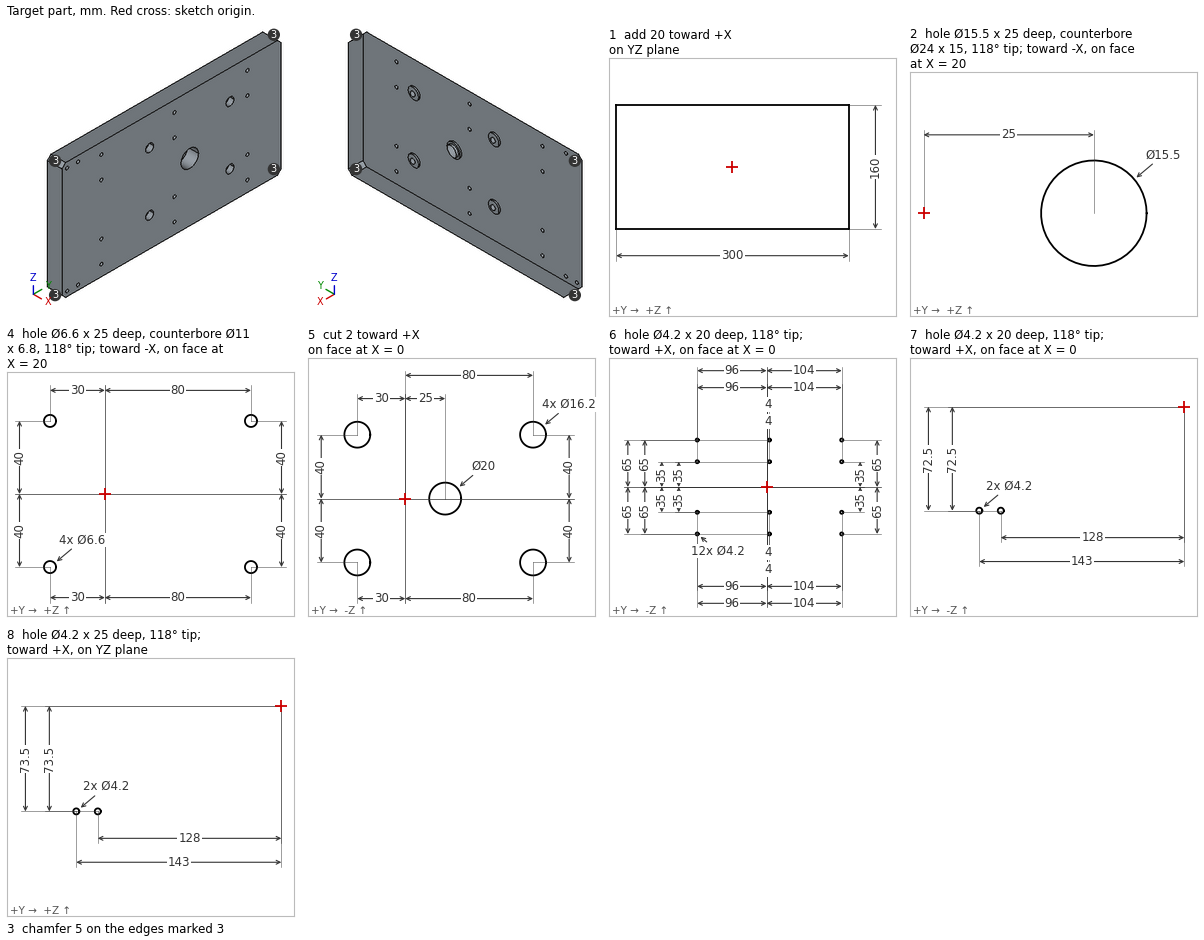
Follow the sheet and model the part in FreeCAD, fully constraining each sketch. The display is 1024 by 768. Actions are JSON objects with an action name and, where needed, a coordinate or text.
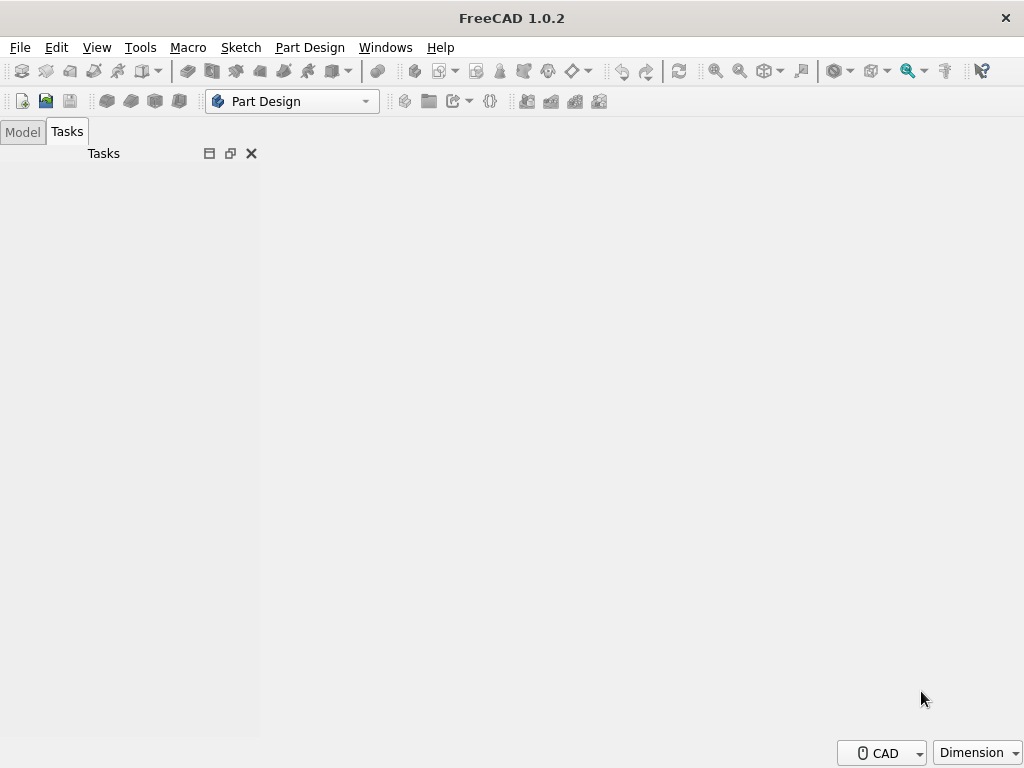
{"action": "left_click", "coordinate": [22, 102]}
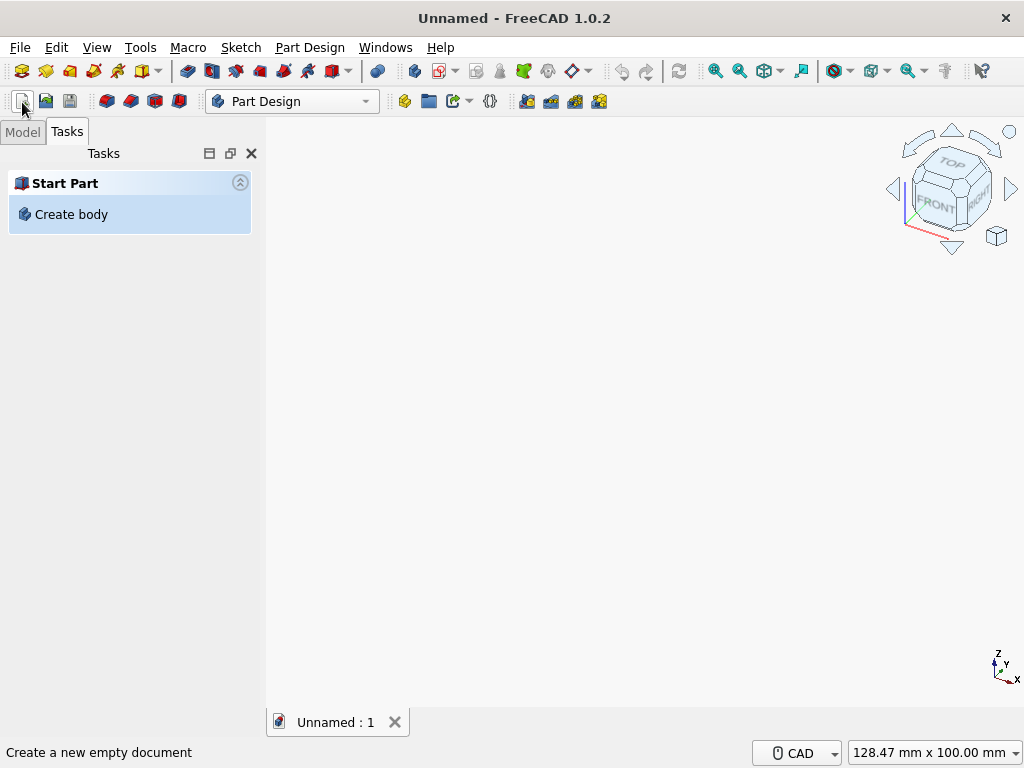
{"action": "left_click", "coordinate": [440, 72]}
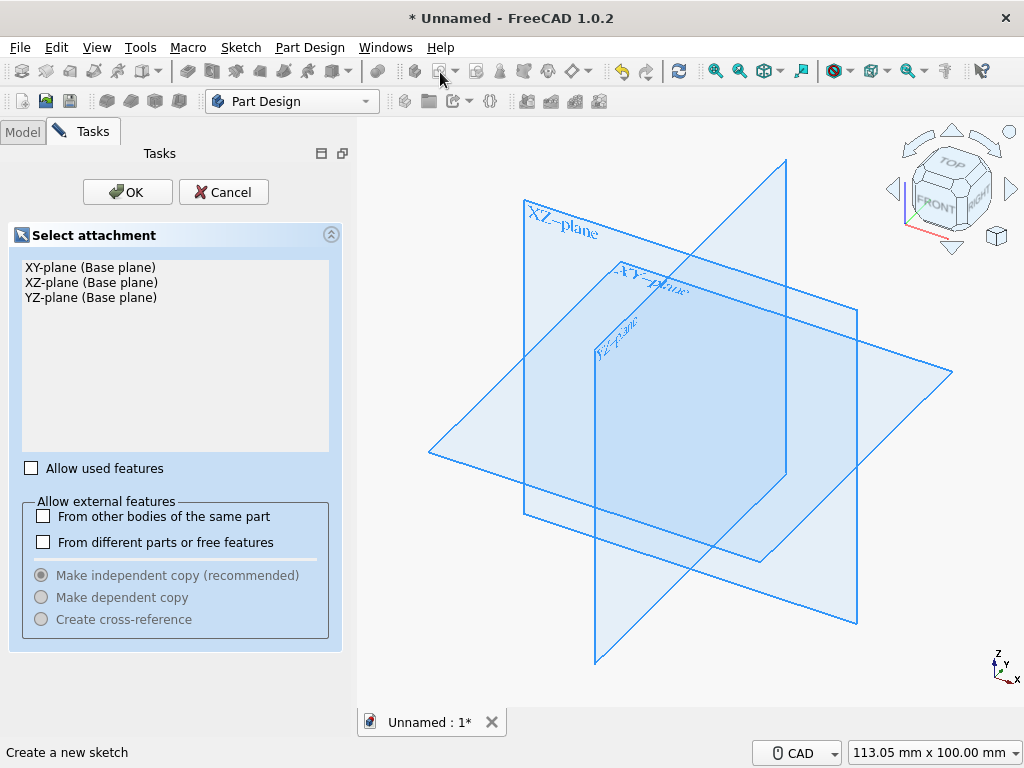
{"action": "left_click", "coordinate": [82, 298]}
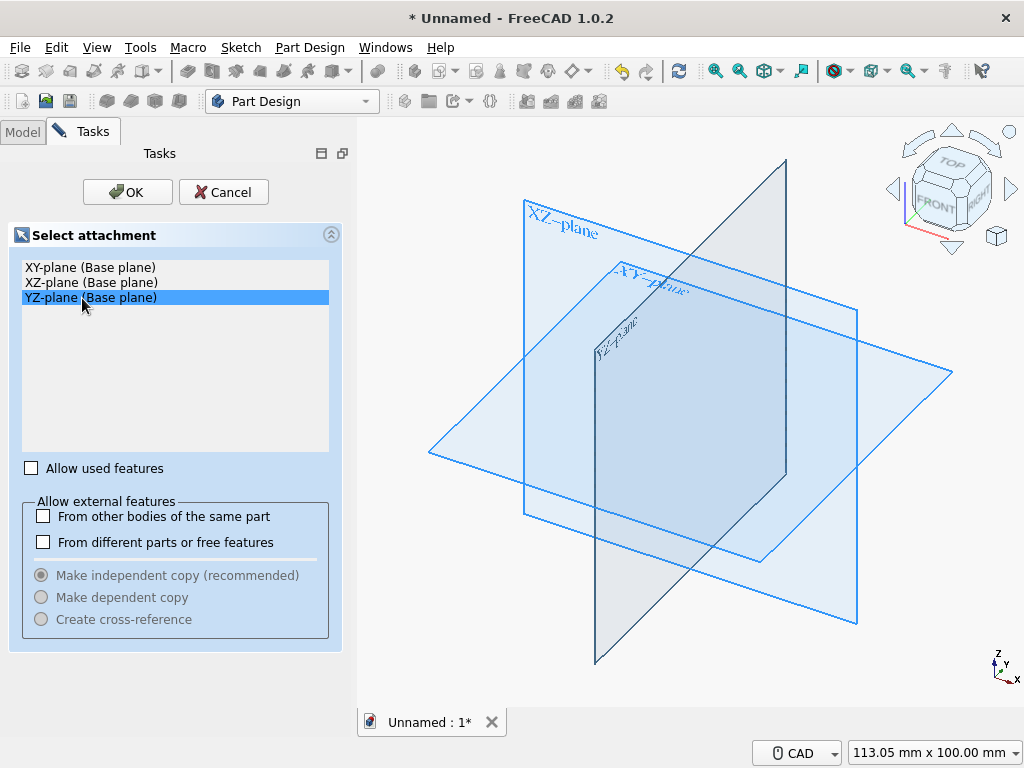
{"action": "left_click", "coordinate": [128, 192]}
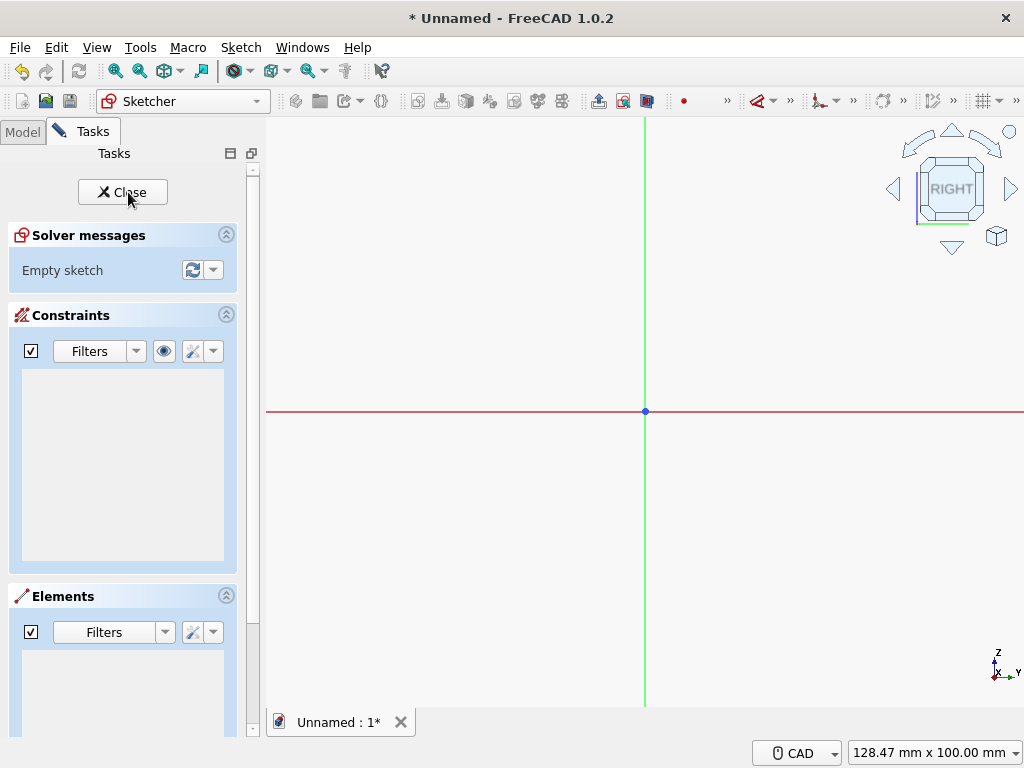
{"action": "scroll", "coordinate": [554, 412], "scroll_direction": "down", "scroll_amount": 7}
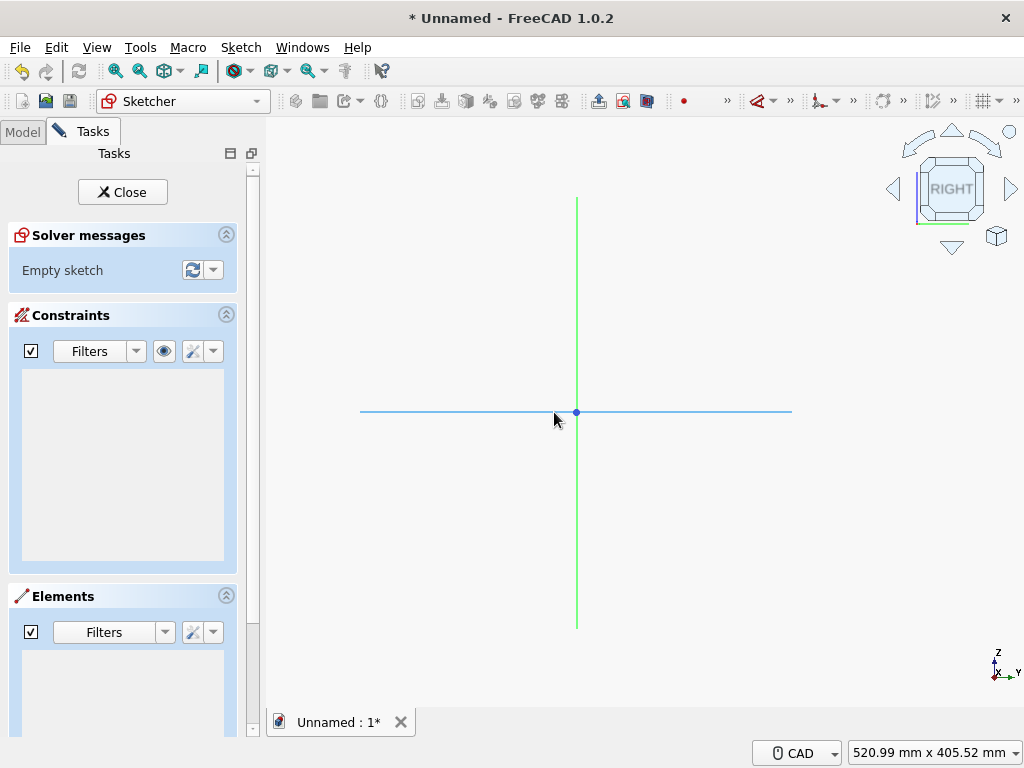
{"action": "key", "text": "g v"}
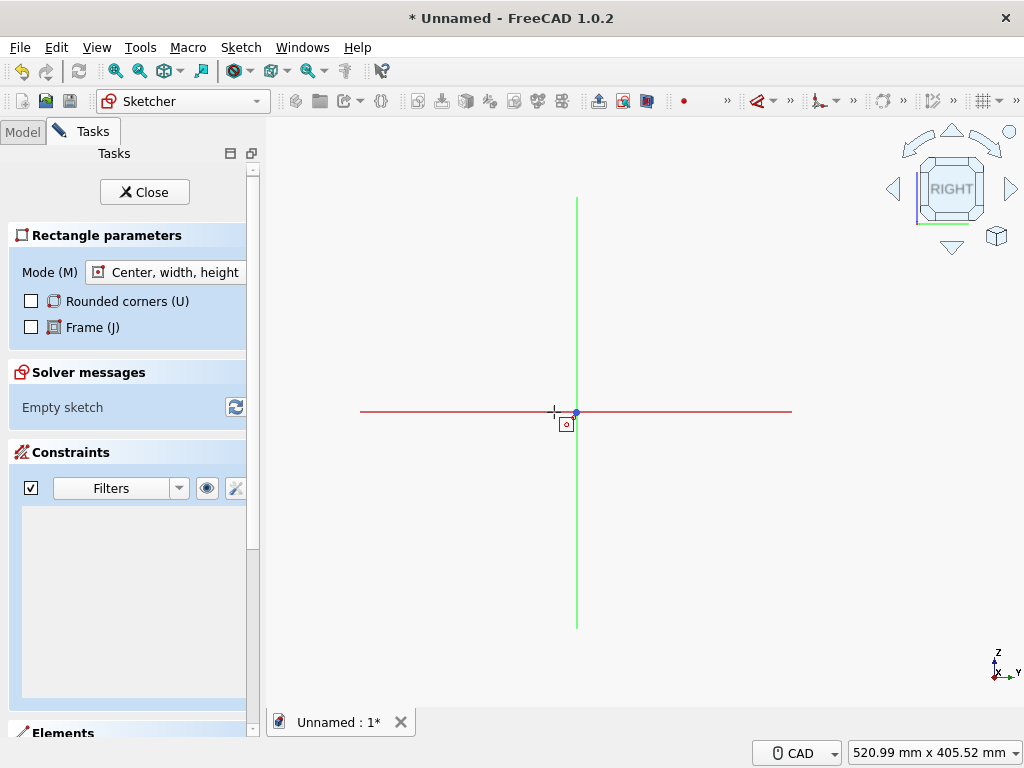
{"action": "left_click", "coordinate": [577, 412]}
{"action": "left_click", "coordinate": [795, 296]}
{"action": "key", "text": "Escape"}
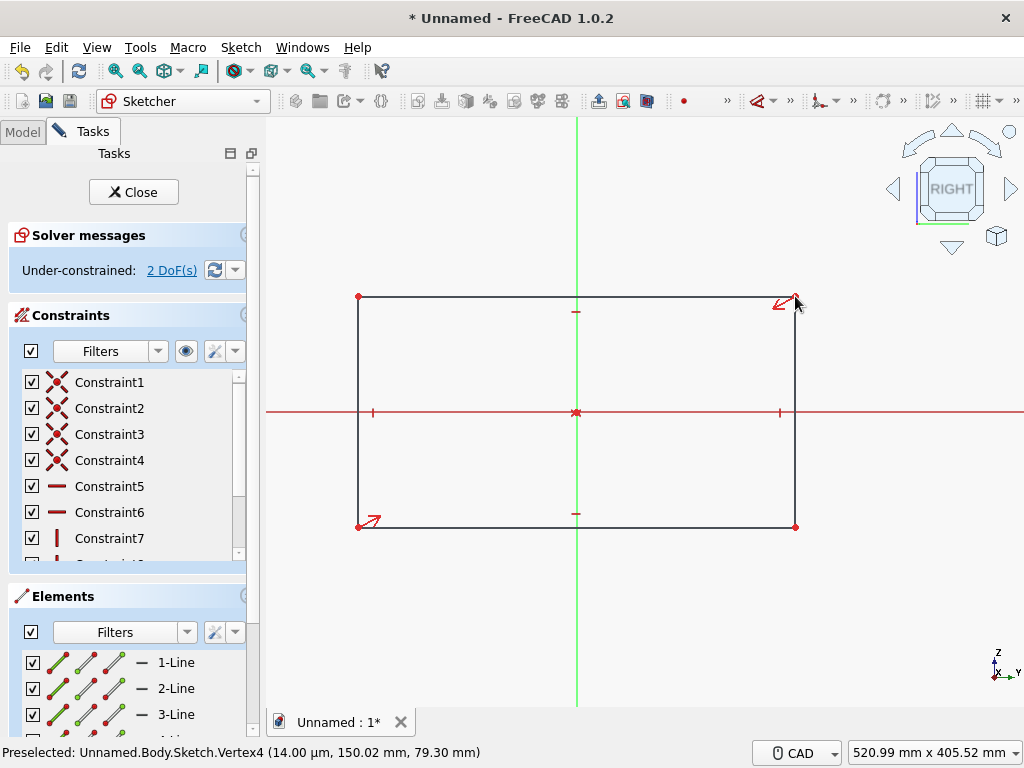
{"action": "key", "text": "d"}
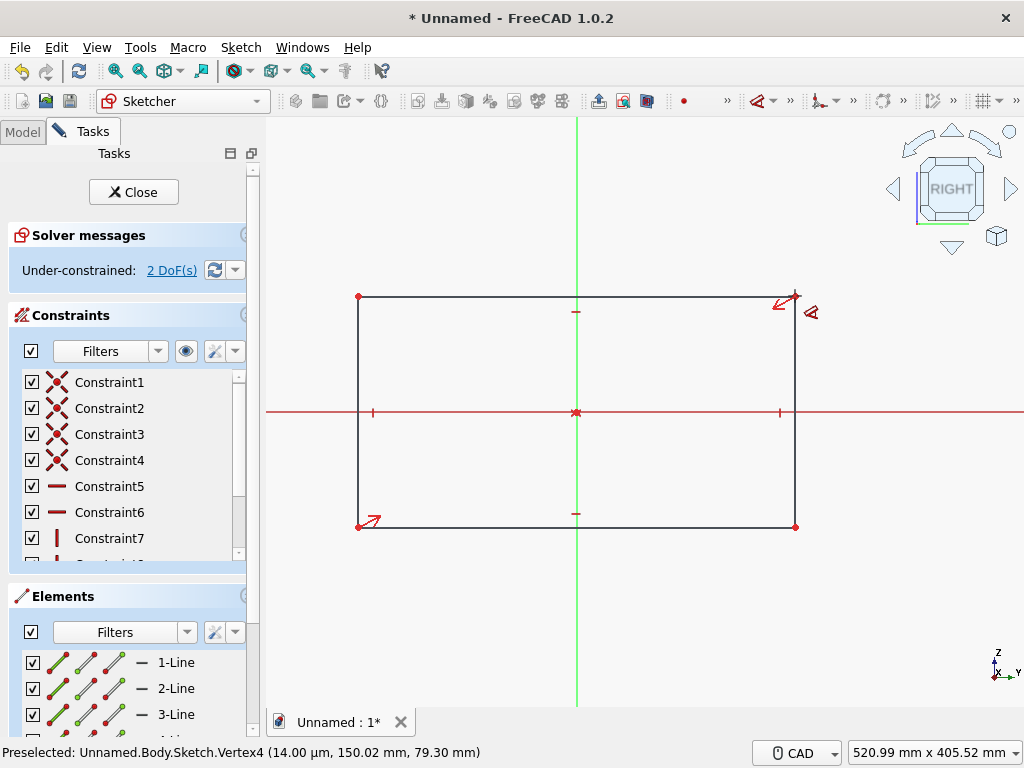
{"action": "left_click", "coordinate": [489, 528]}
{"action": "left_click", "coordinate": [476, 562]}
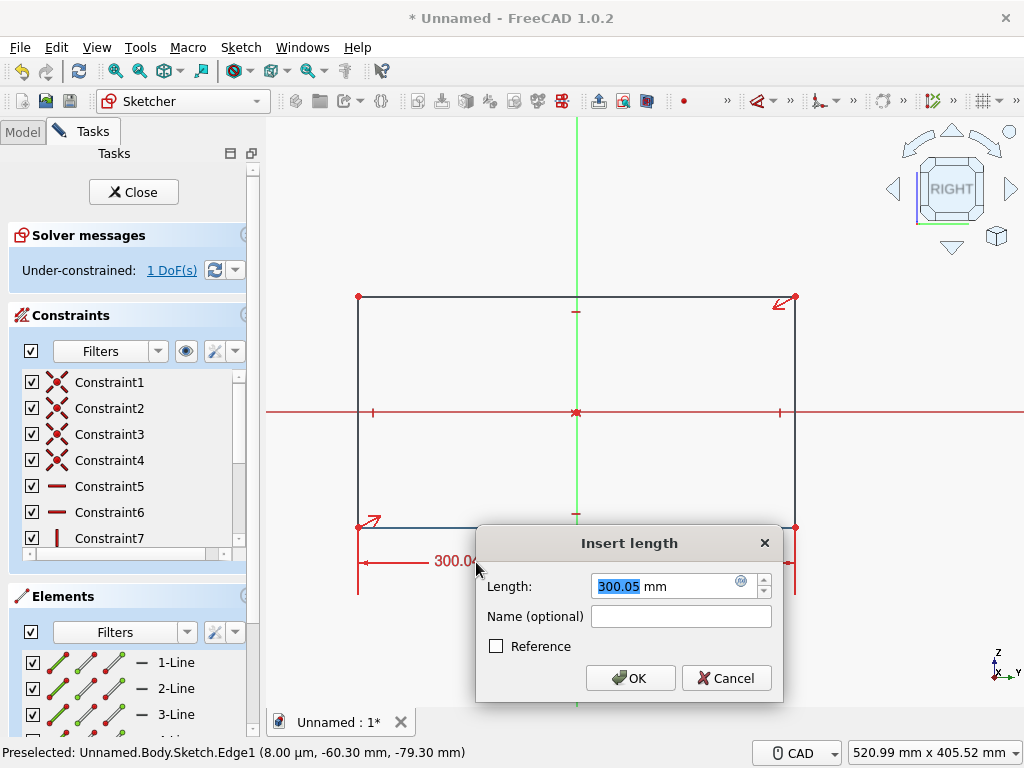
{"action": "type", "text": "300"}
{"action": "key", "text": "Return"}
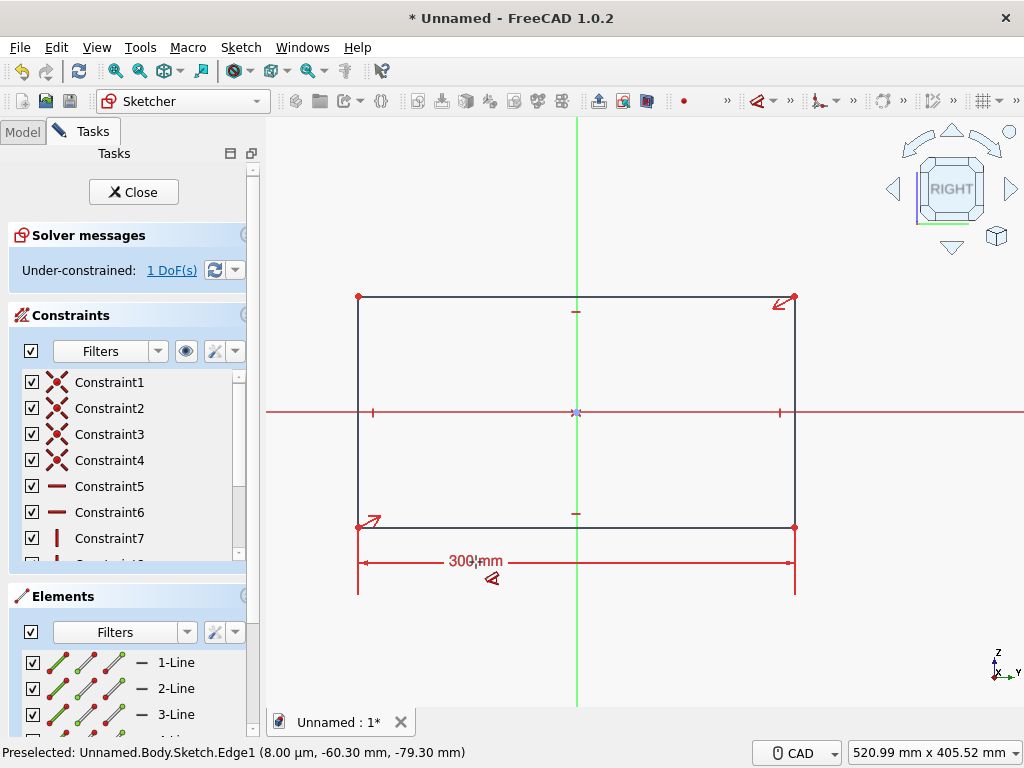
{"action": "left_click", "coordinate": [795, 459]}
{"action": "left_click", "coordinate": [829, 359]}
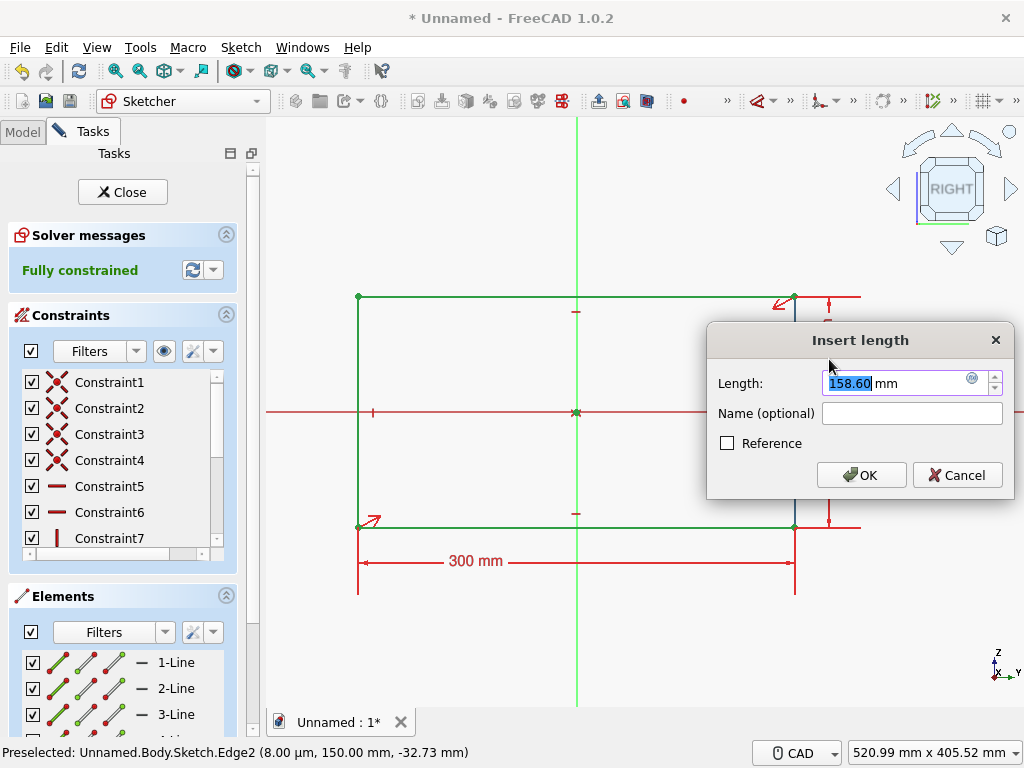
{"action": "type", "text": "160"}
{"action": "key", "text": "Return"}
{"action": "key", "text": "Escape"}